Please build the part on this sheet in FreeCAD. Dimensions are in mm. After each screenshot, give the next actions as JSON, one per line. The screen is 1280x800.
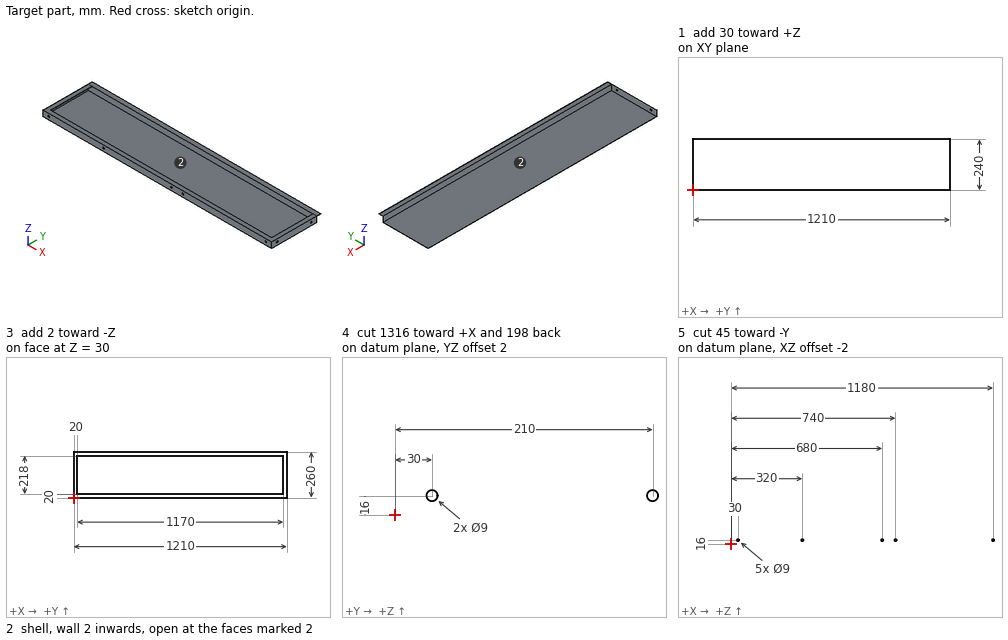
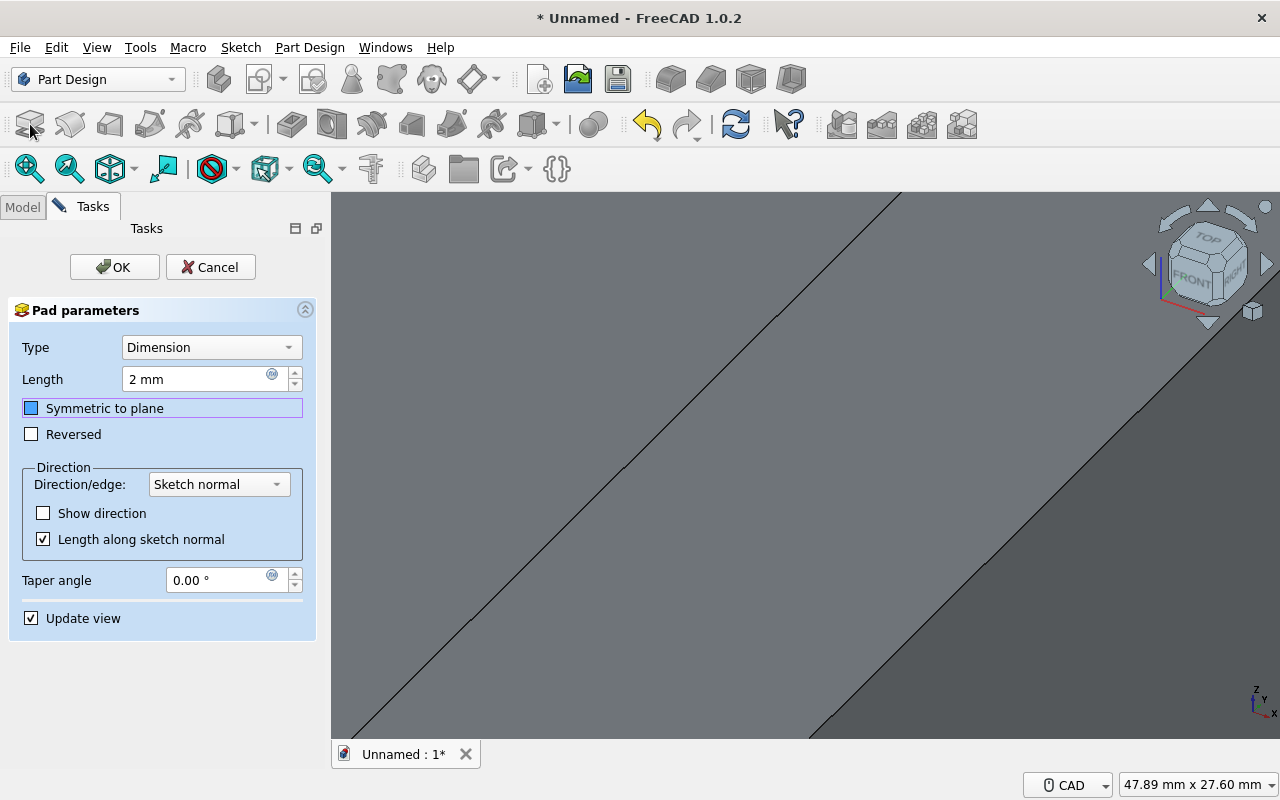
{"action": "left_click", "coordinate": [30, 434]}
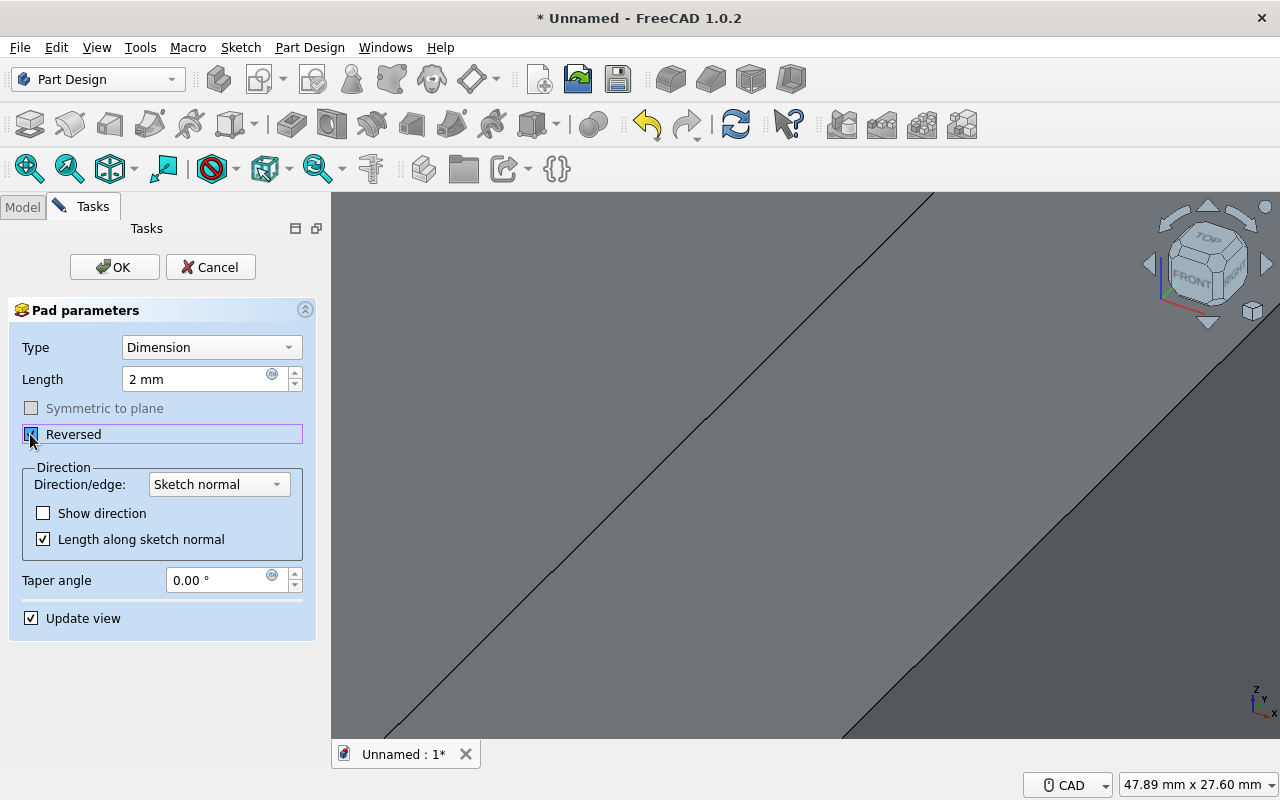
{"action": "left_click", "coordinate": [115, 267]}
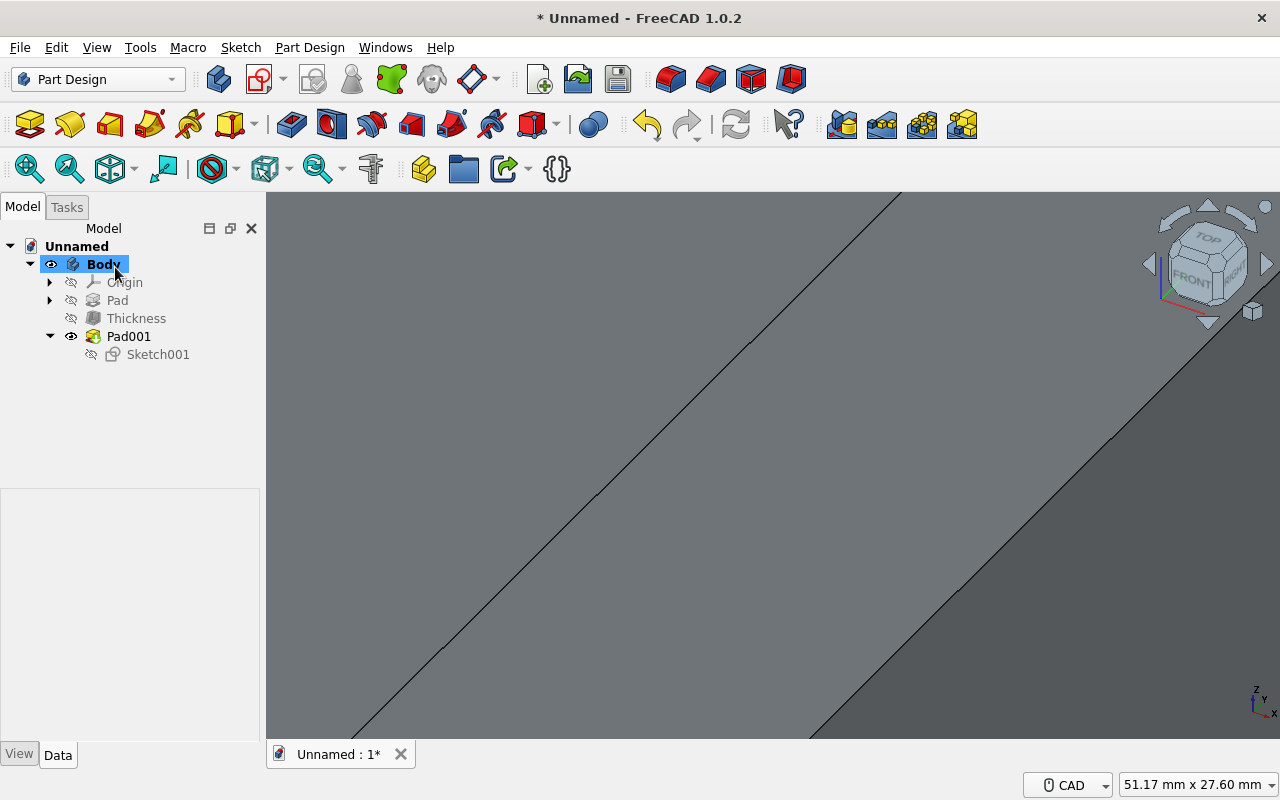
{"action": "left_click", "coordinate": [30, 170]}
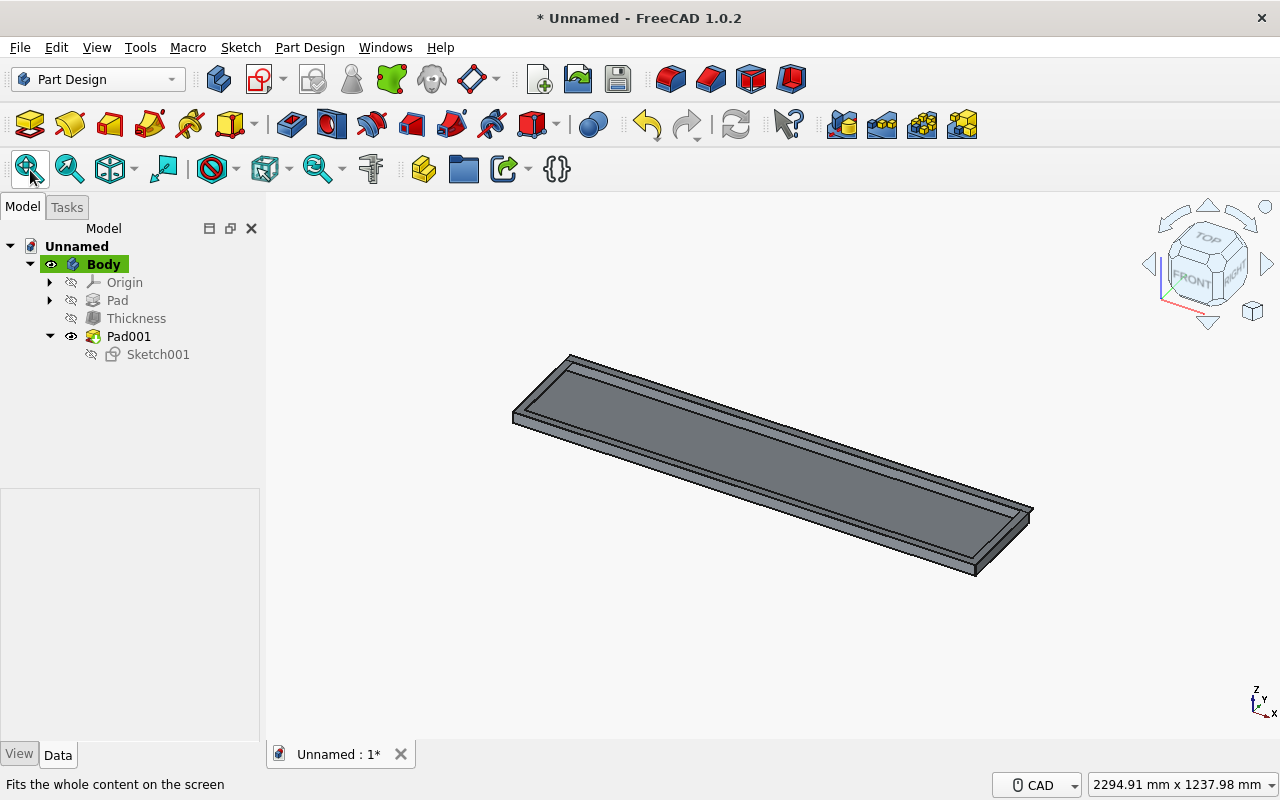
{"action": "left_click", "coordinate": [50, 282]}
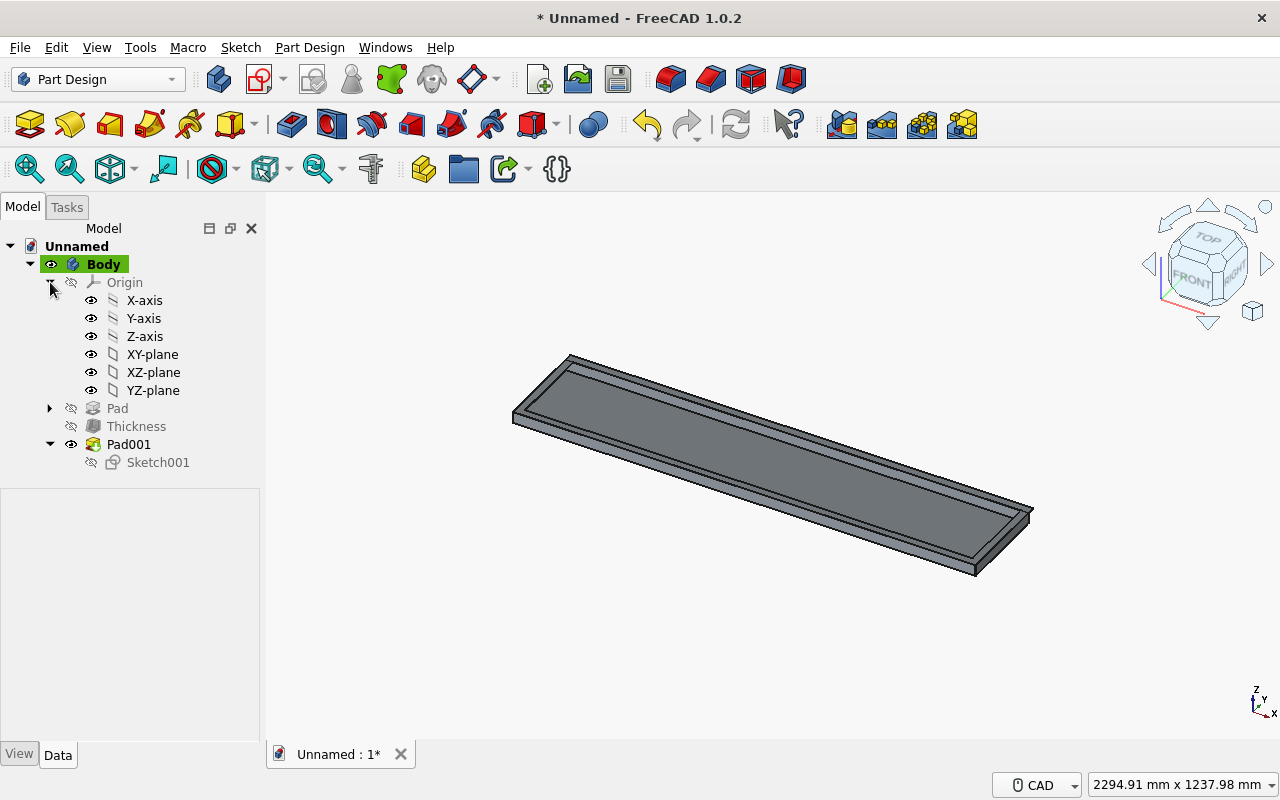
{"action": "left_click", "coordinate": [136, 390]}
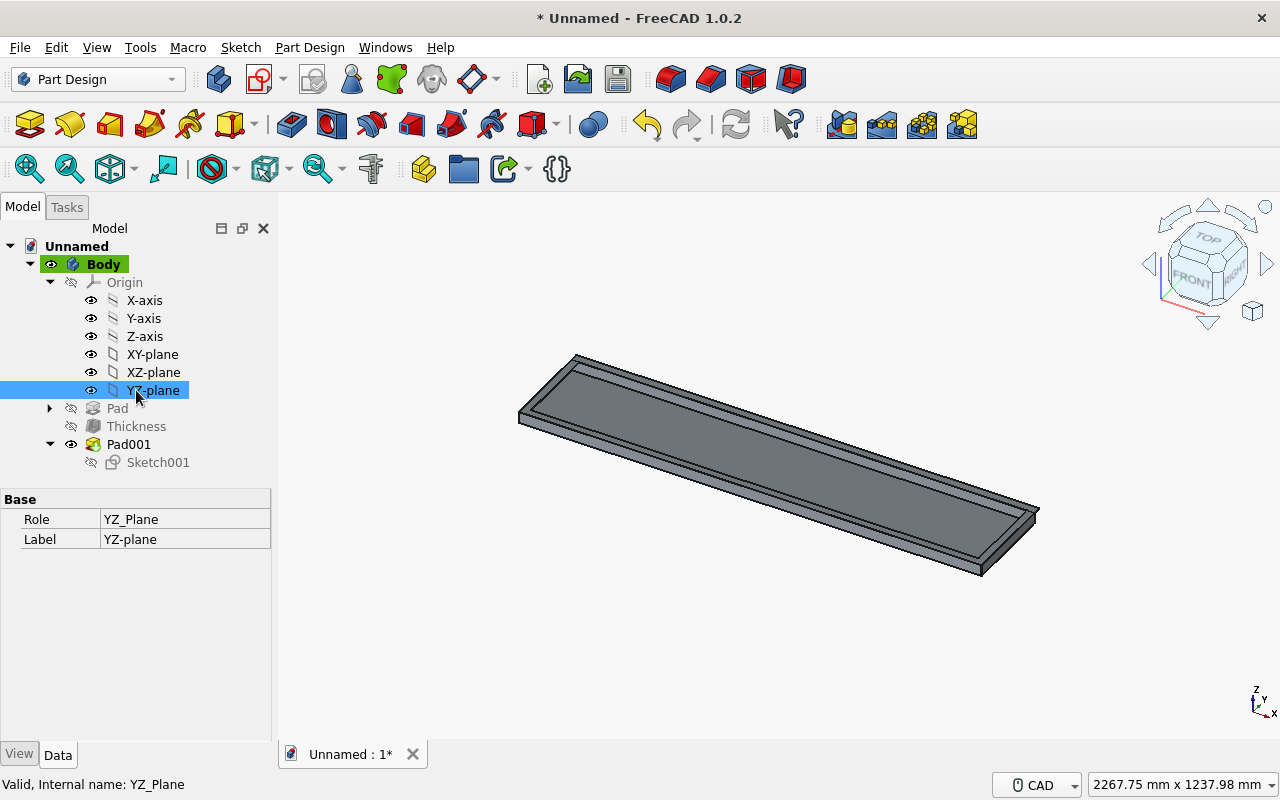
{"action": "left_click", "coordinate": [472, 80]}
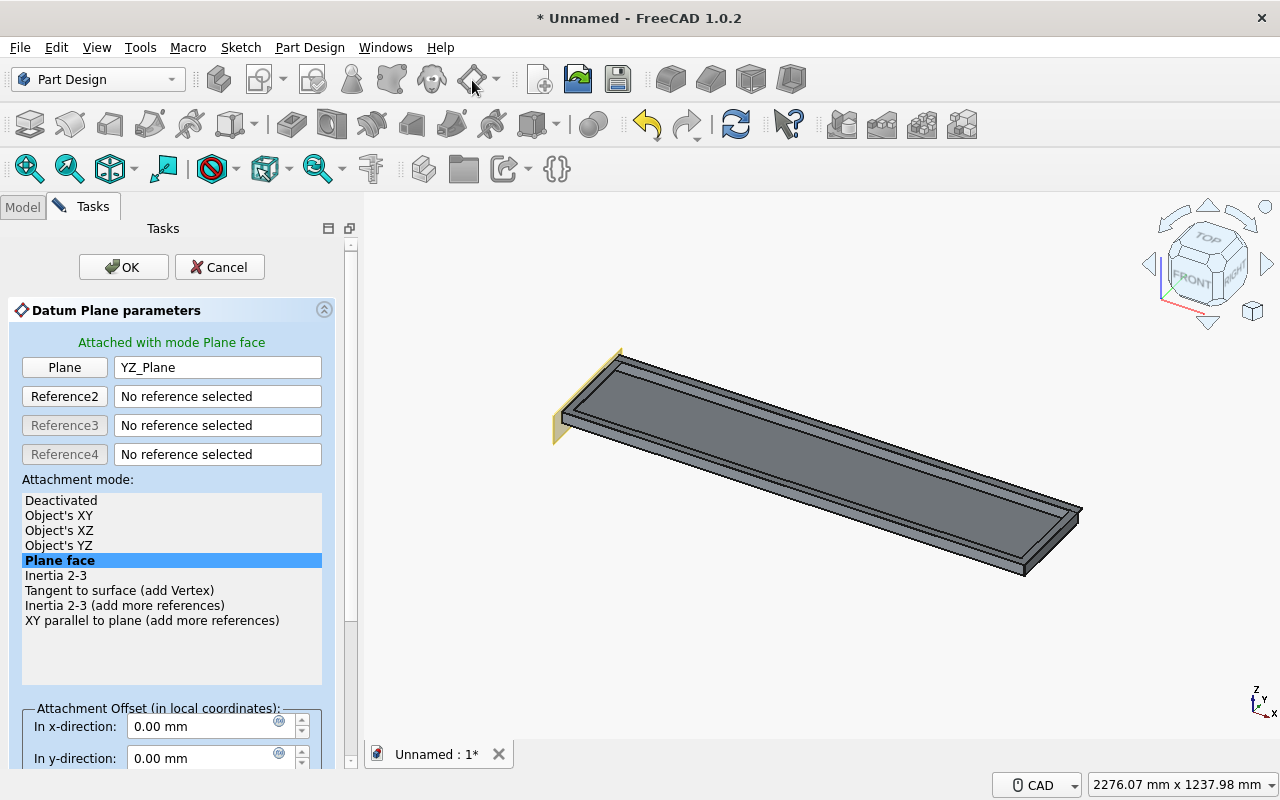
{"action": "scroll", "coordinate": [351, 503], "scroll_direction": "down", "scroll_amount": 2}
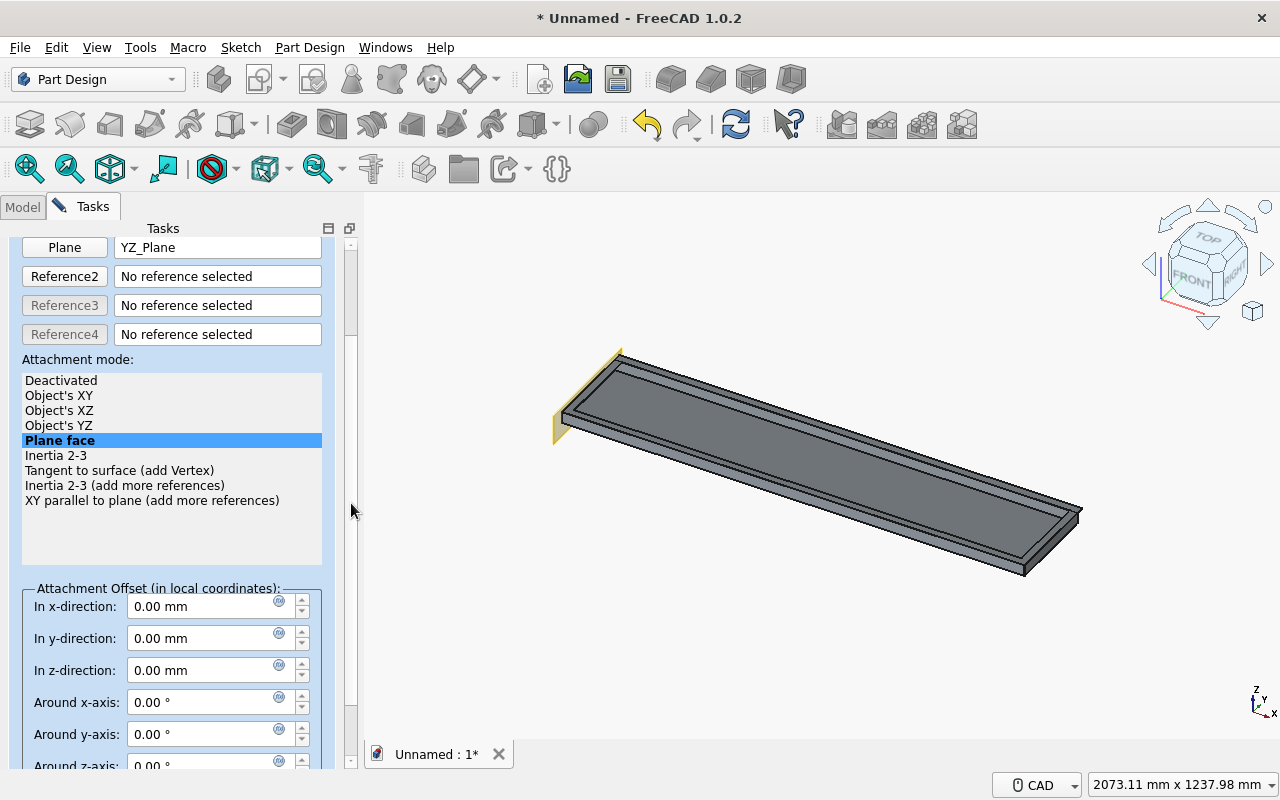
{"action": "triple_click", "coordinate": [210, 670]}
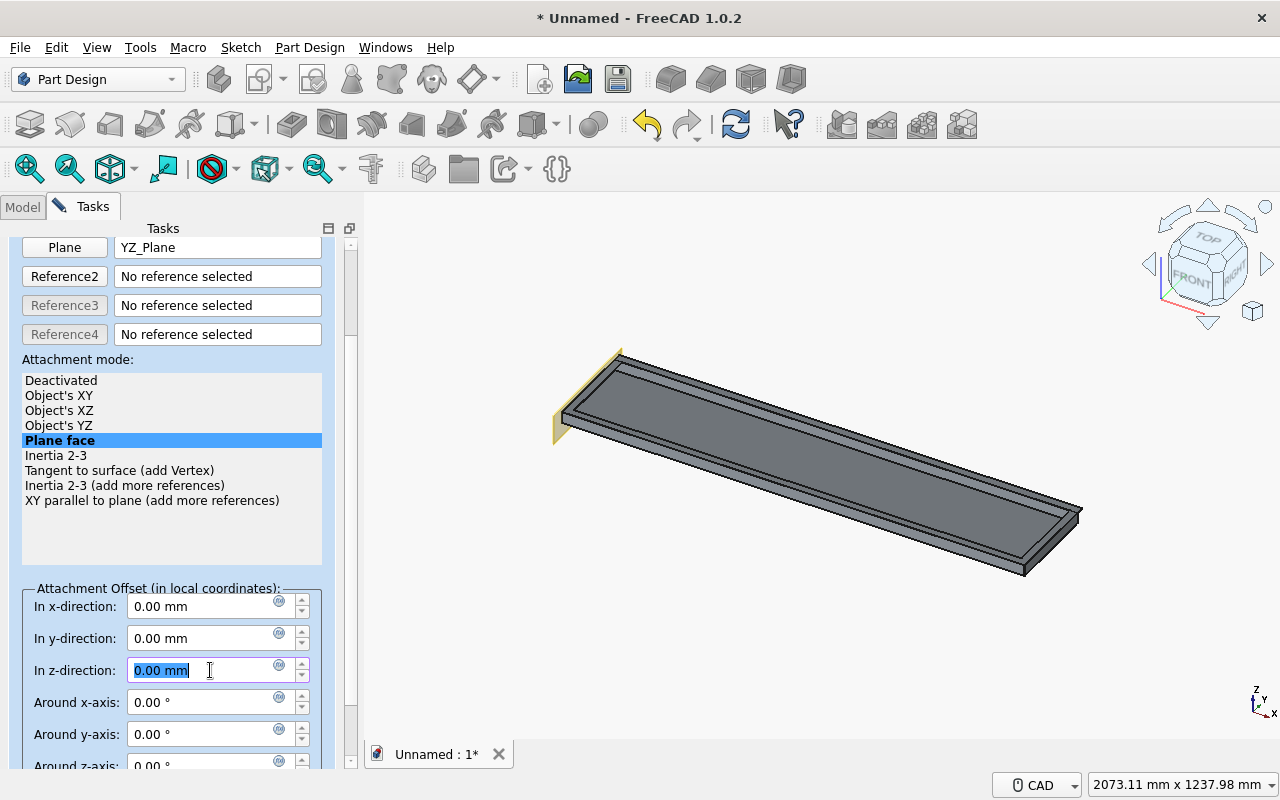
{"action": "type", "text": "2"}
{"action": "key", "text": "Tab"}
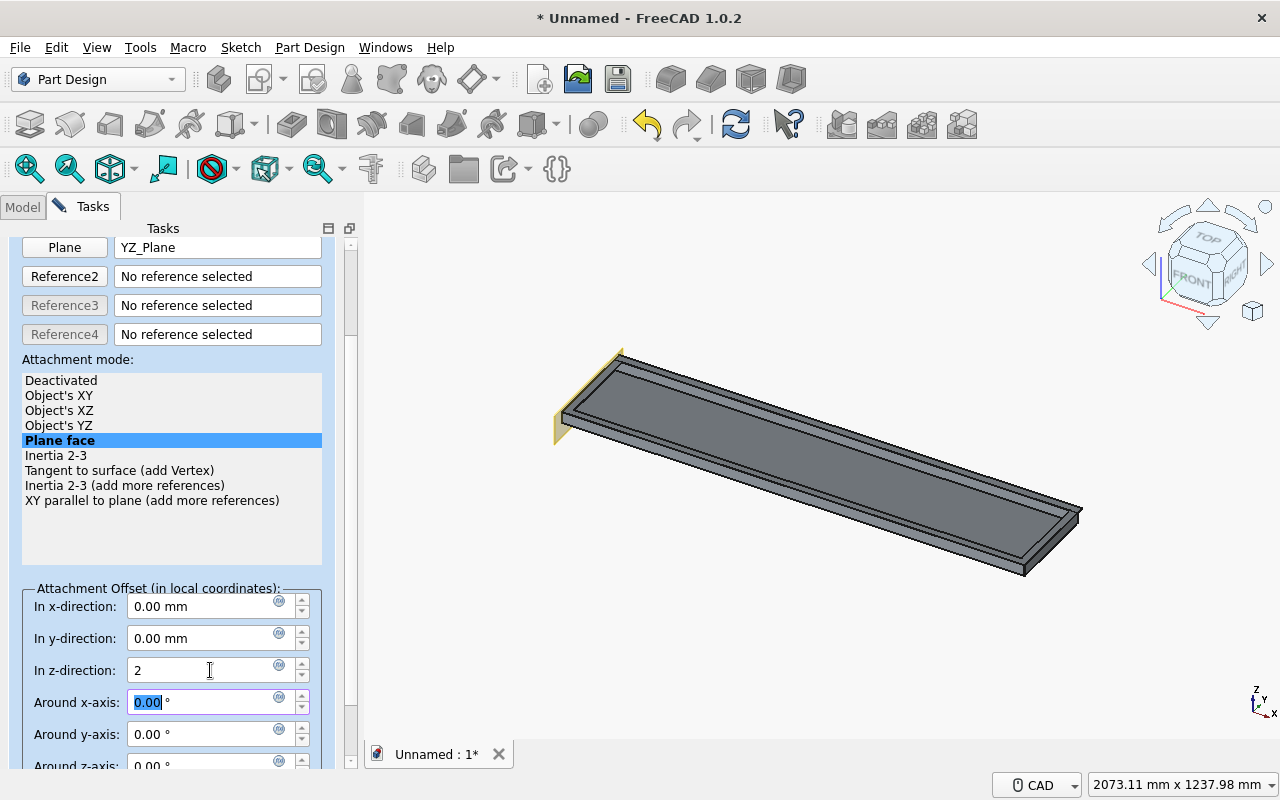
{"action": "scroll", "coordinate": [351, 503], "scroll_direction": "up", "scroll_amount": 3}